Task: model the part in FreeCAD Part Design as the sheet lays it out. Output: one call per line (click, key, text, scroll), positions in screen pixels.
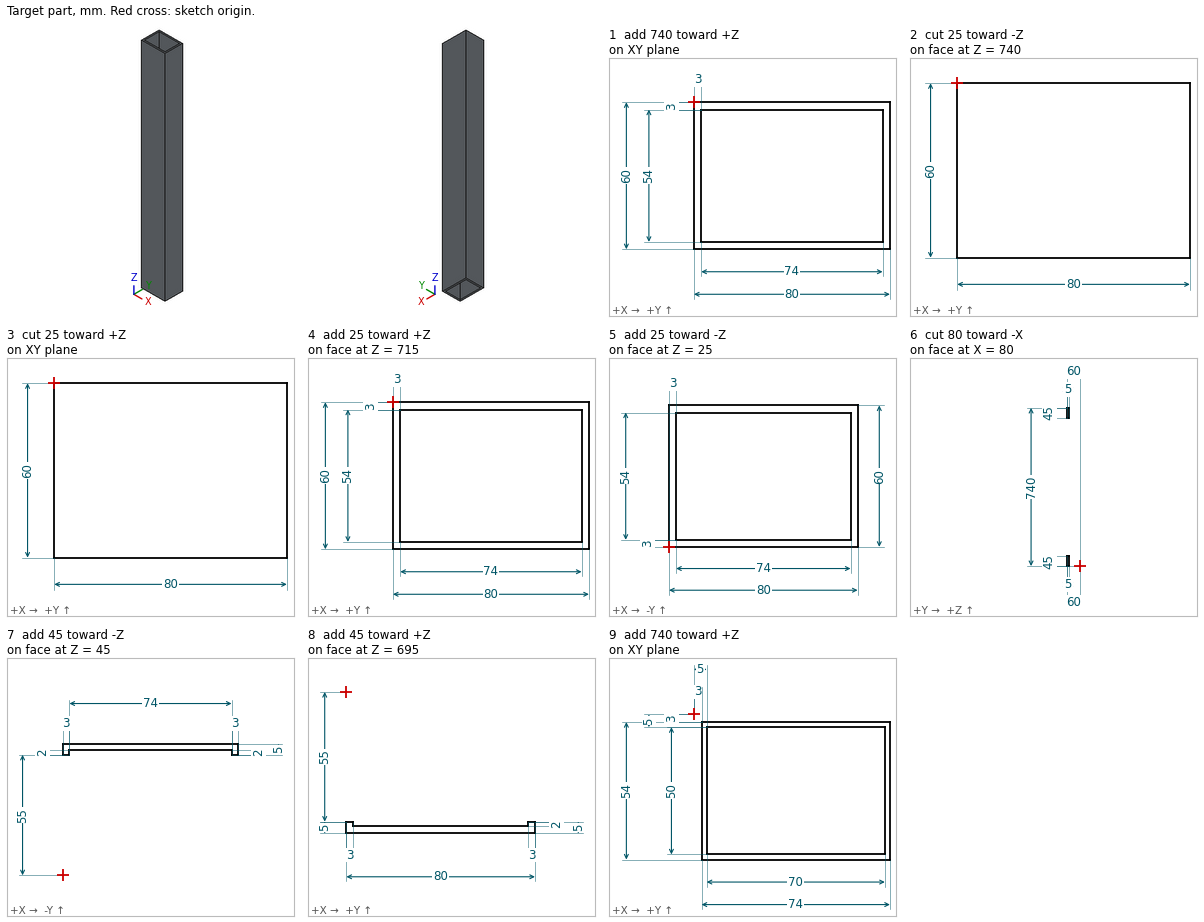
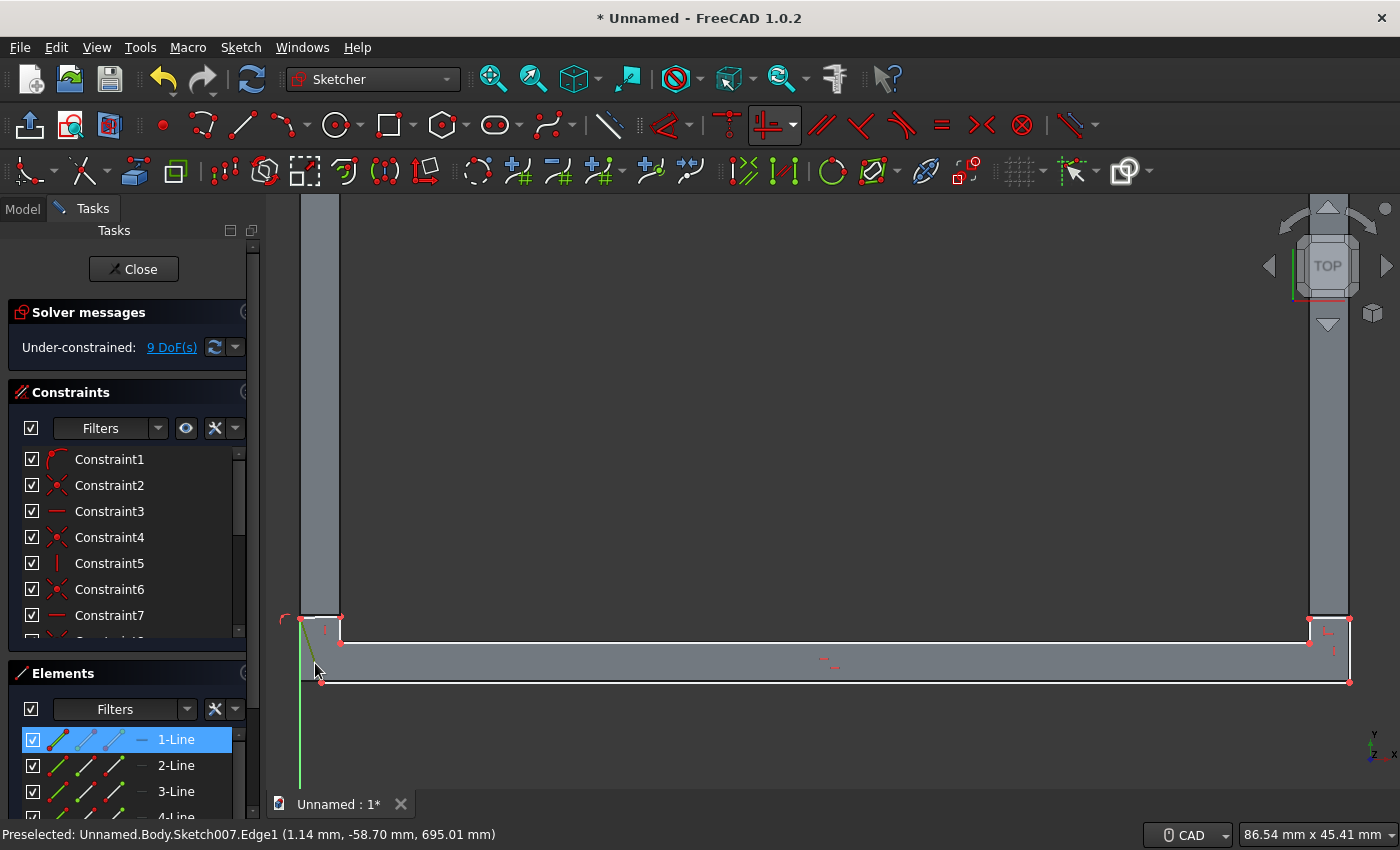
key(v)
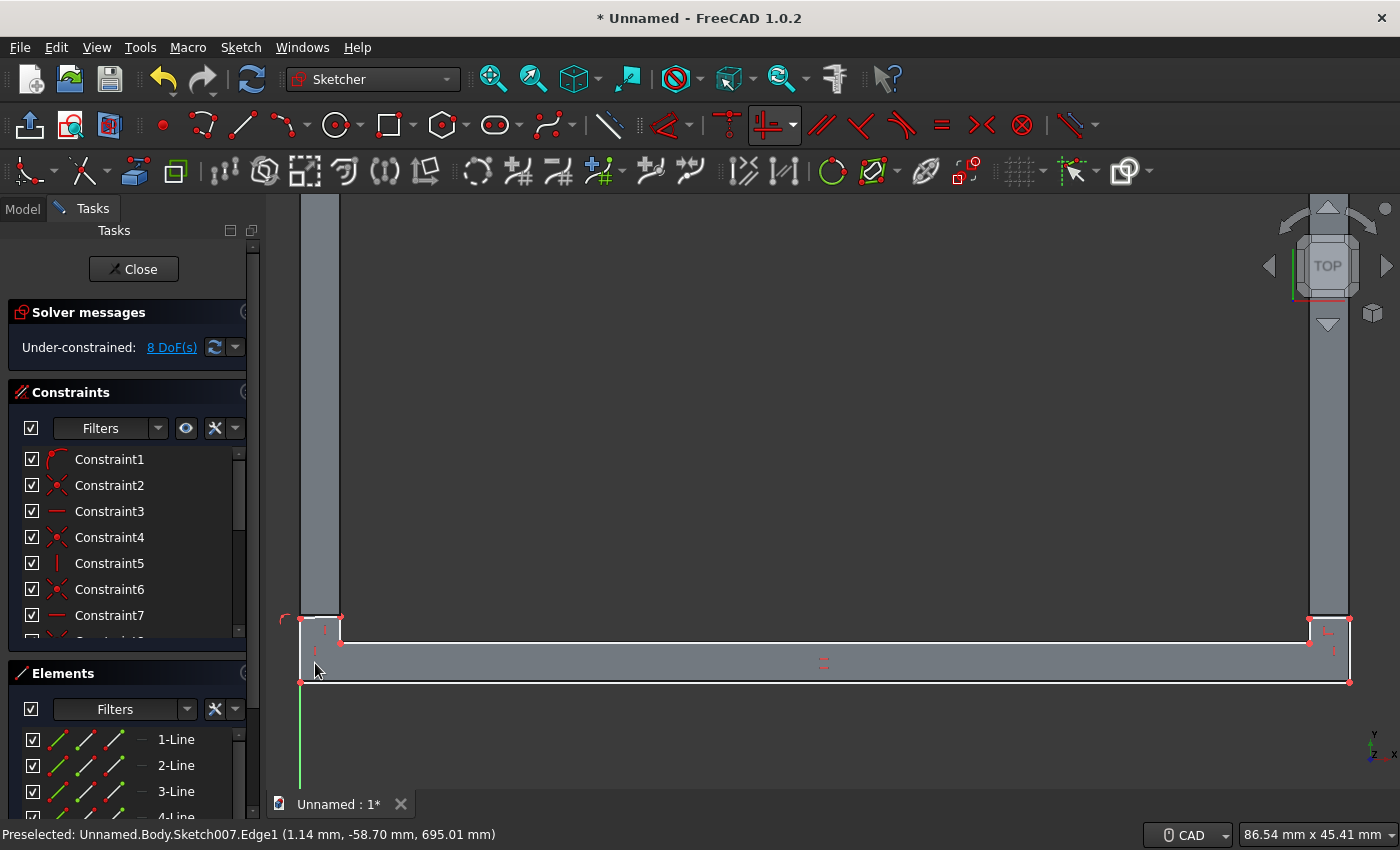
click(328, 617)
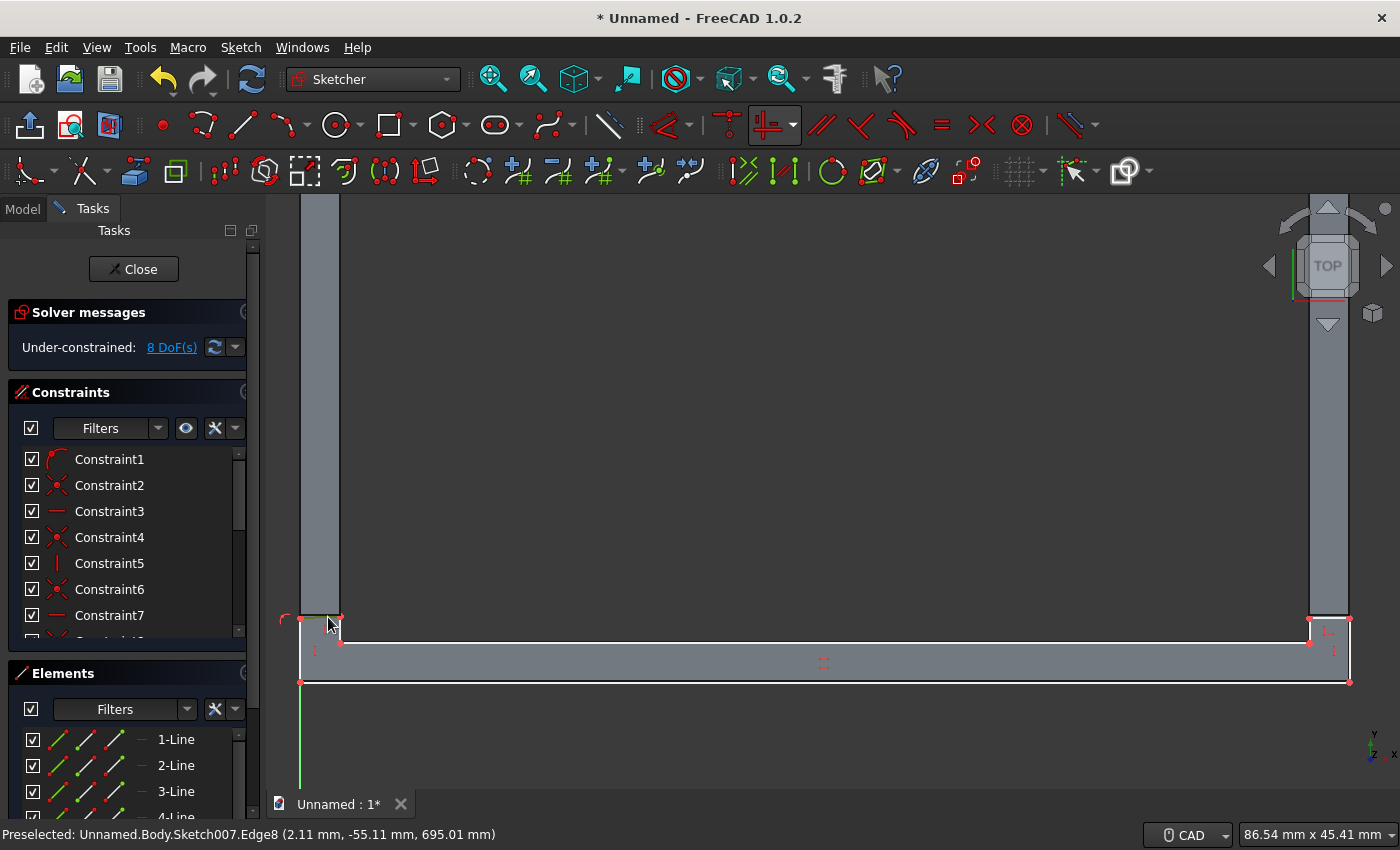
key(h)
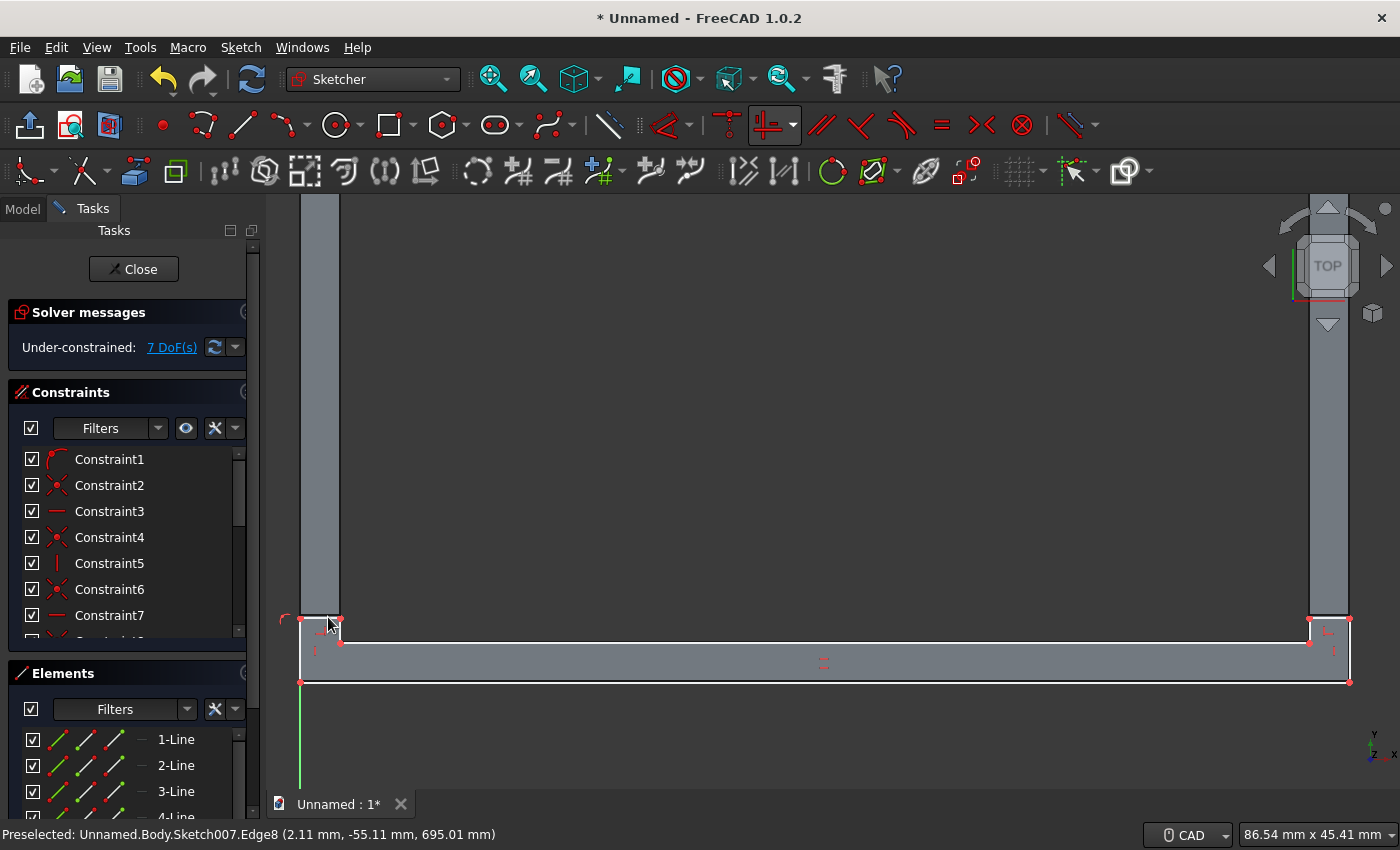
key(d)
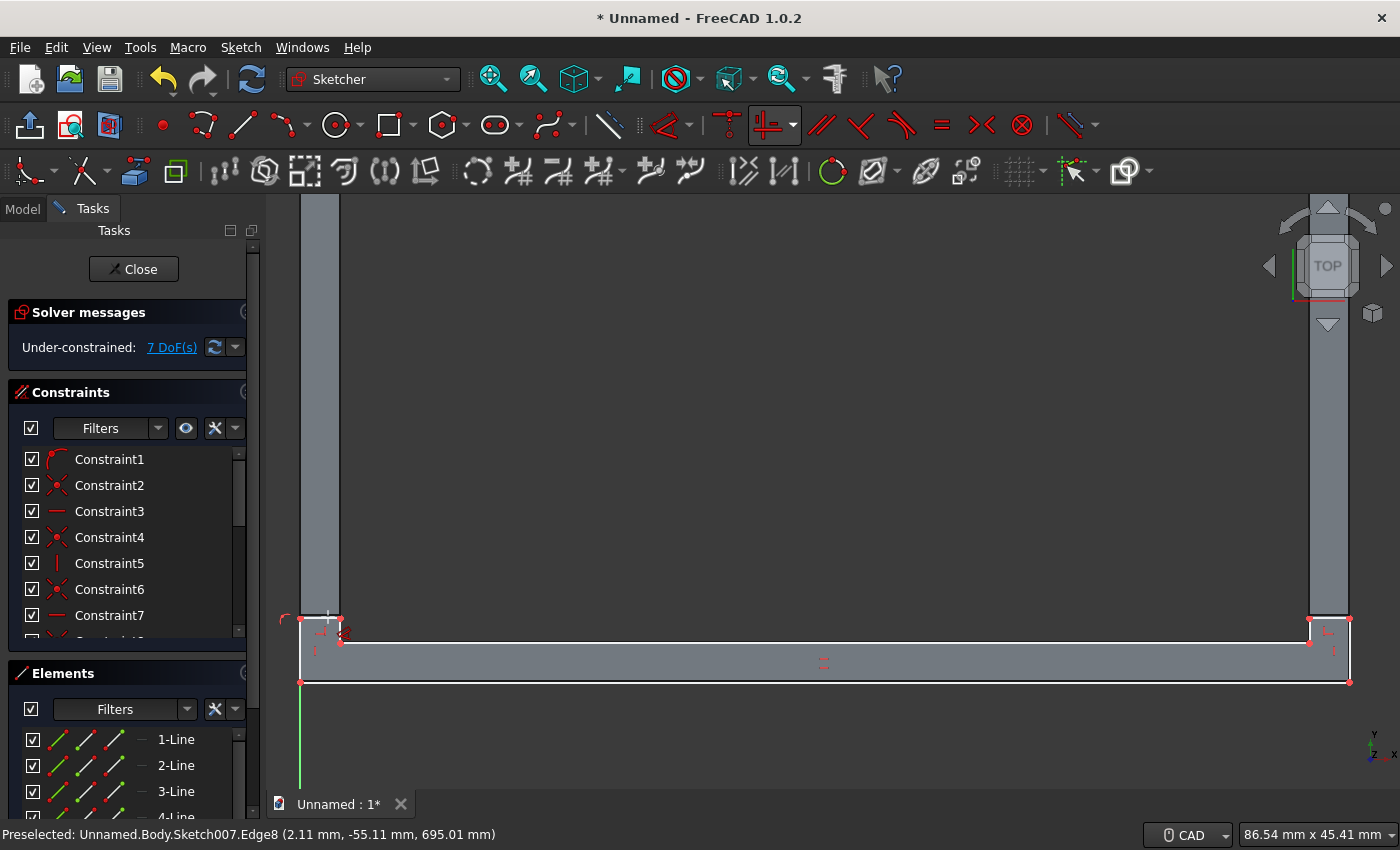
click(300, 638)
click(334, 665)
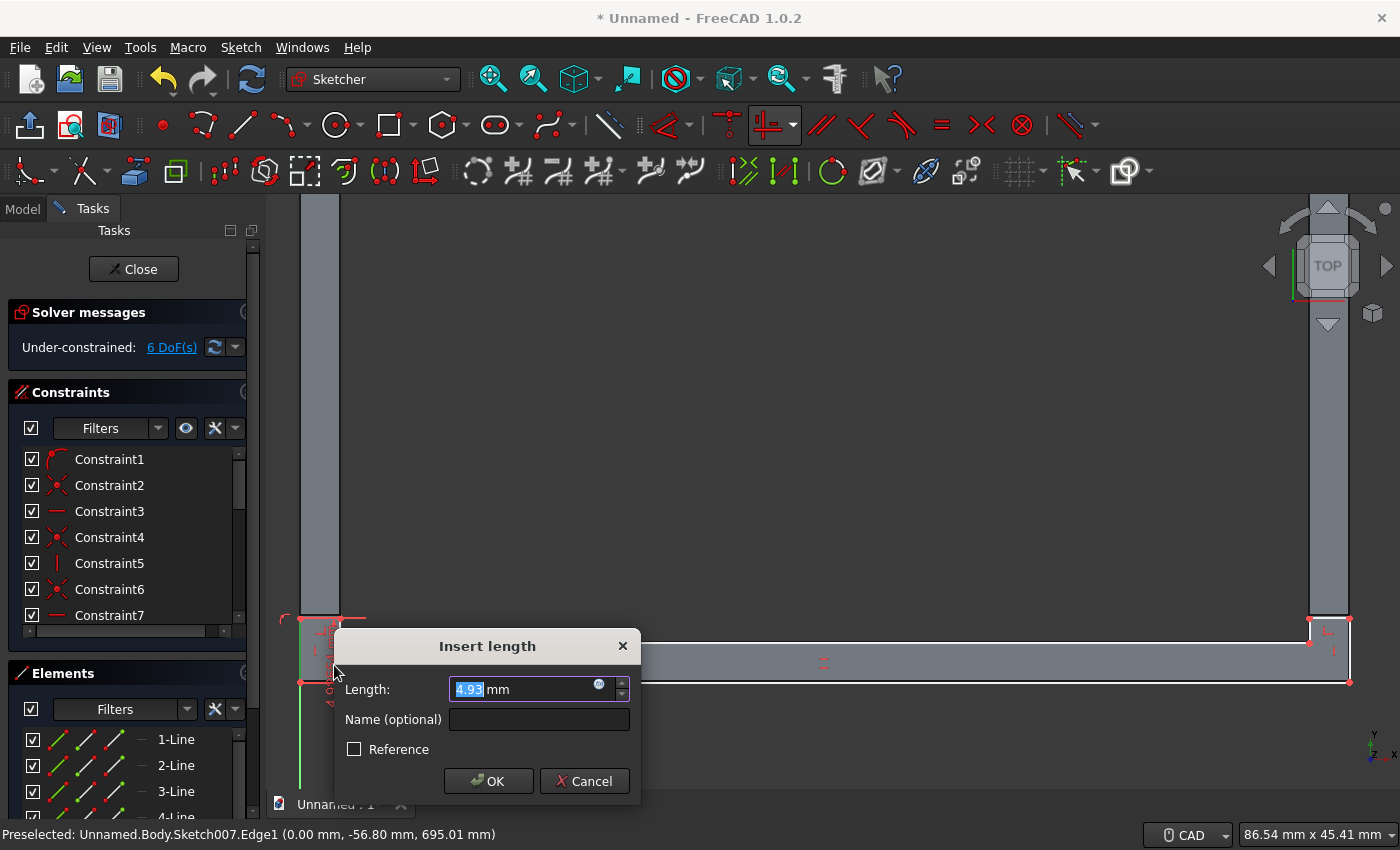
text(5)
key(Return)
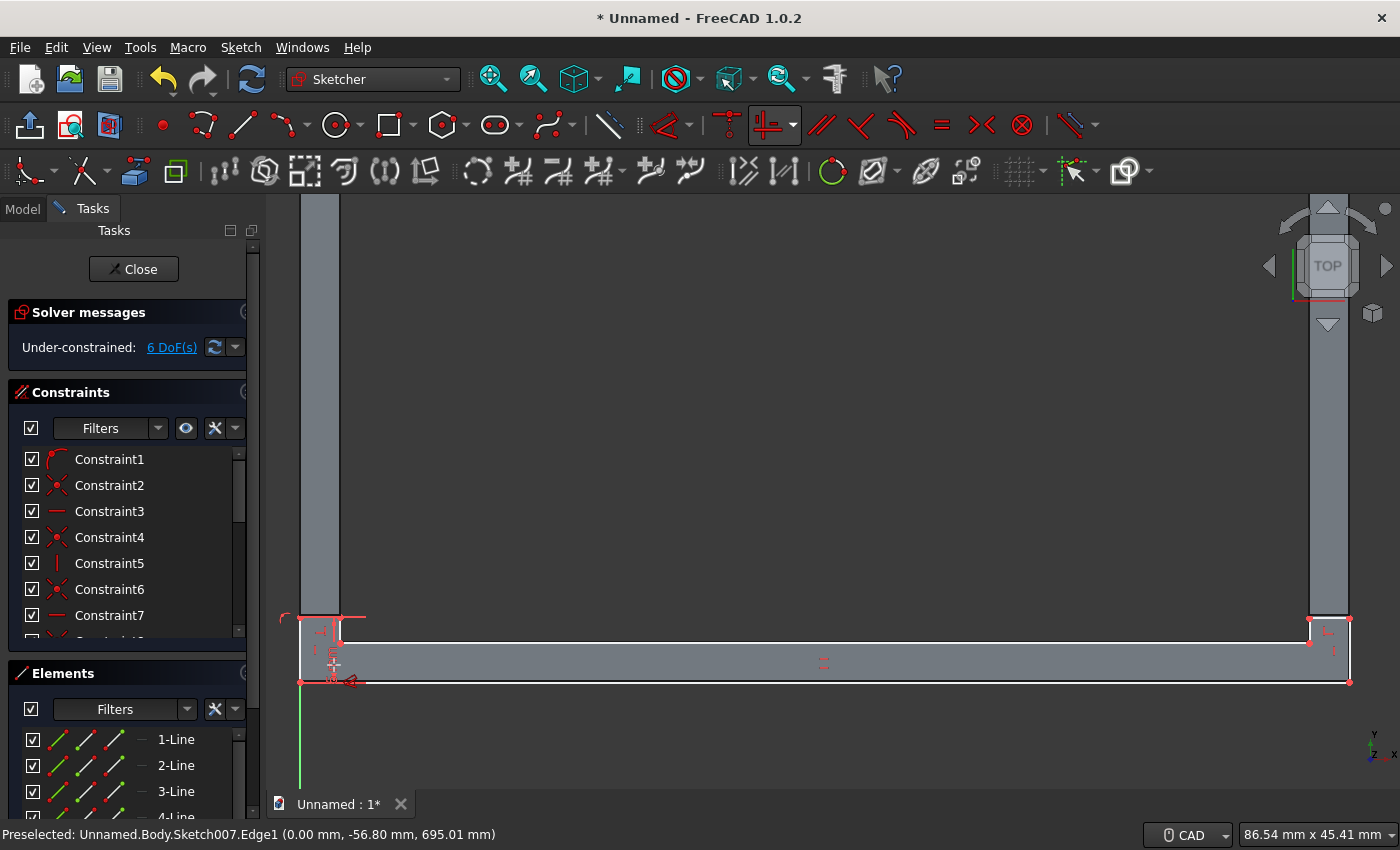
scroll(716, 658, down, 4)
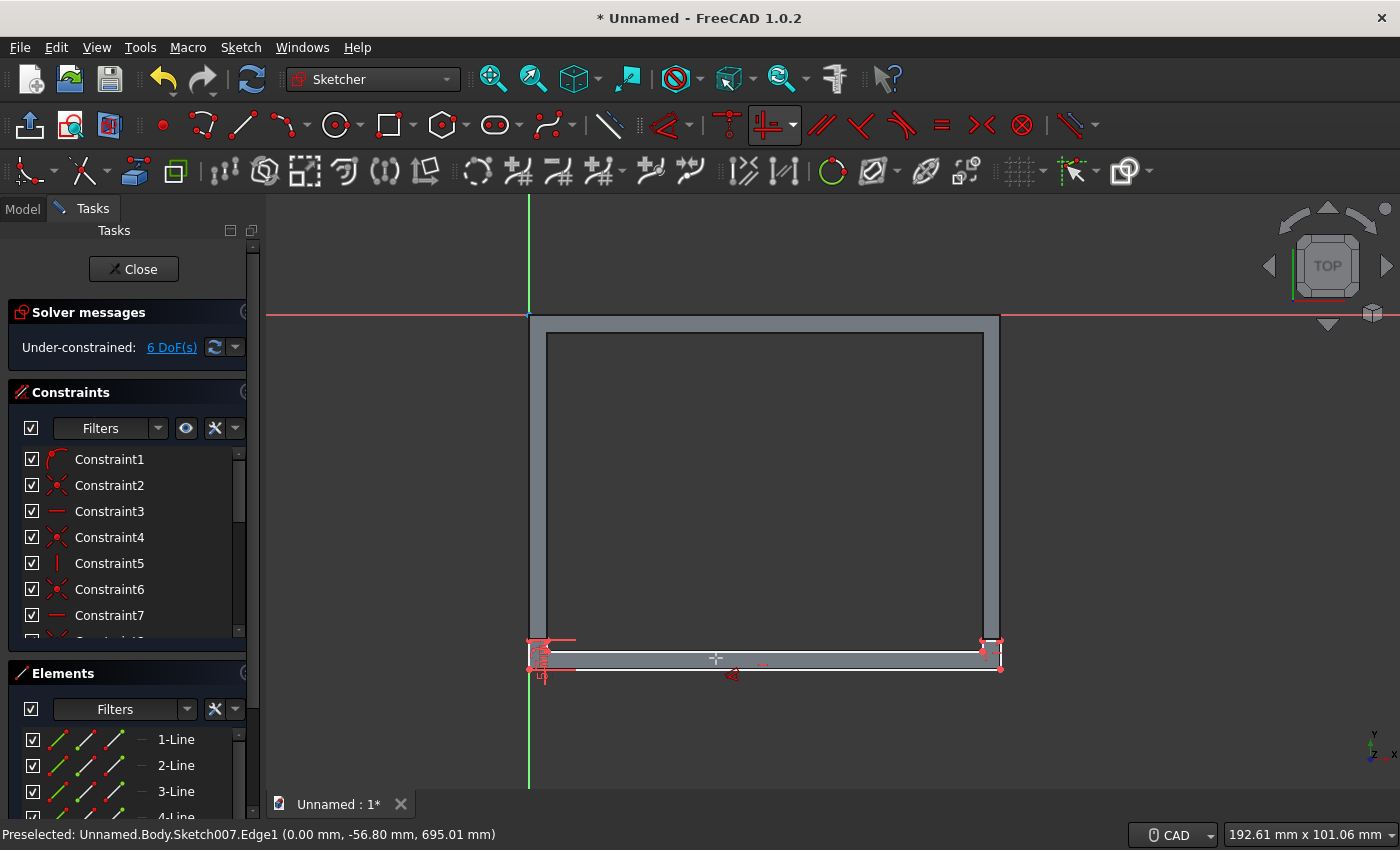
scroll(1001, 661, up, 3)